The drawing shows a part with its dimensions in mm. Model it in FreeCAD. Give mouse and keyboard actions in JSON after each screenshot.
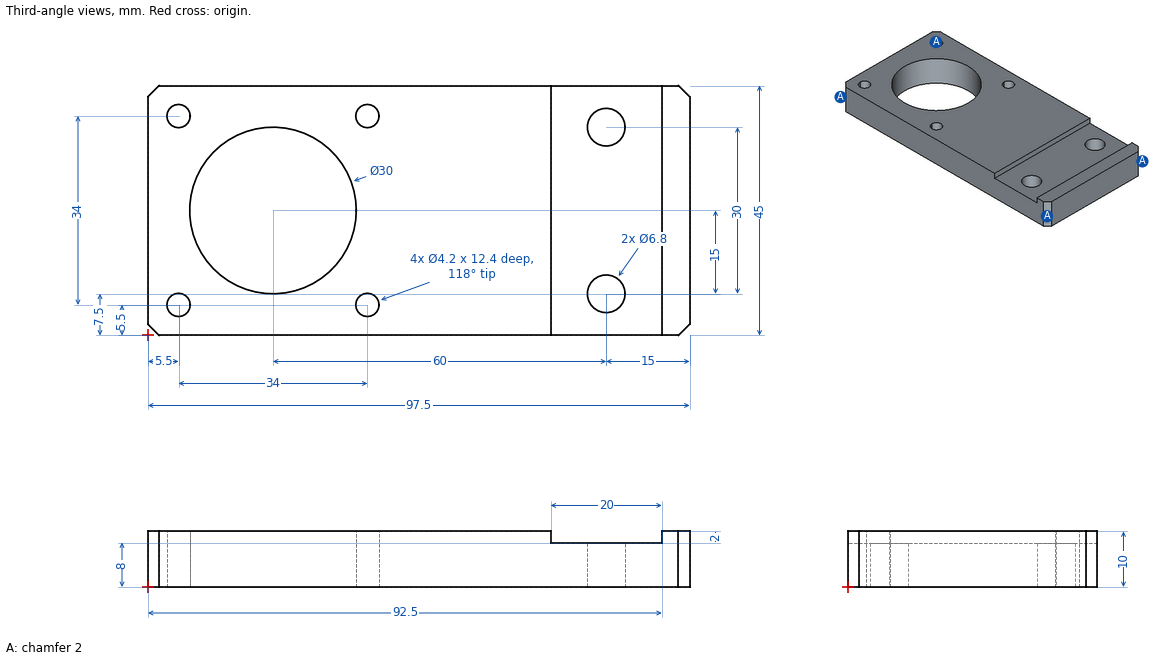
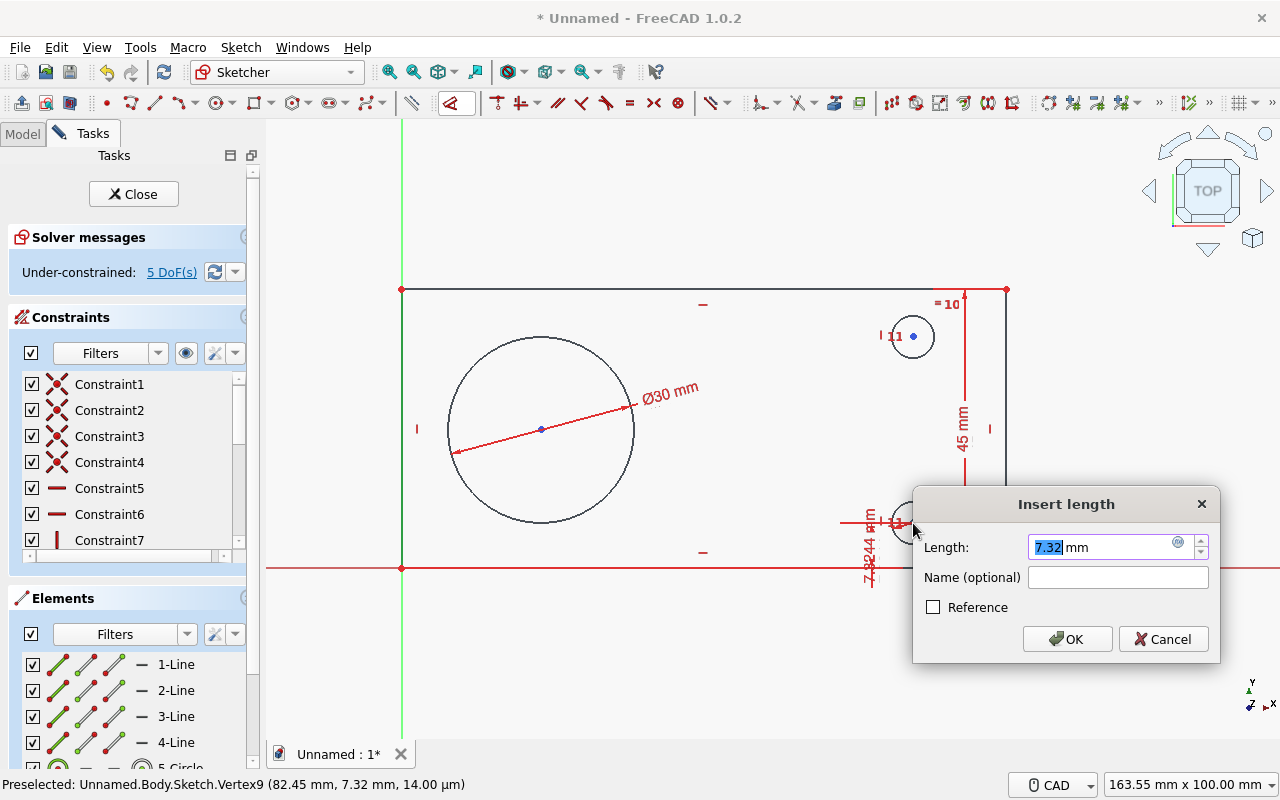
{"action": "type", "text": "7.5"}
{"action": "key", "text": "Return"}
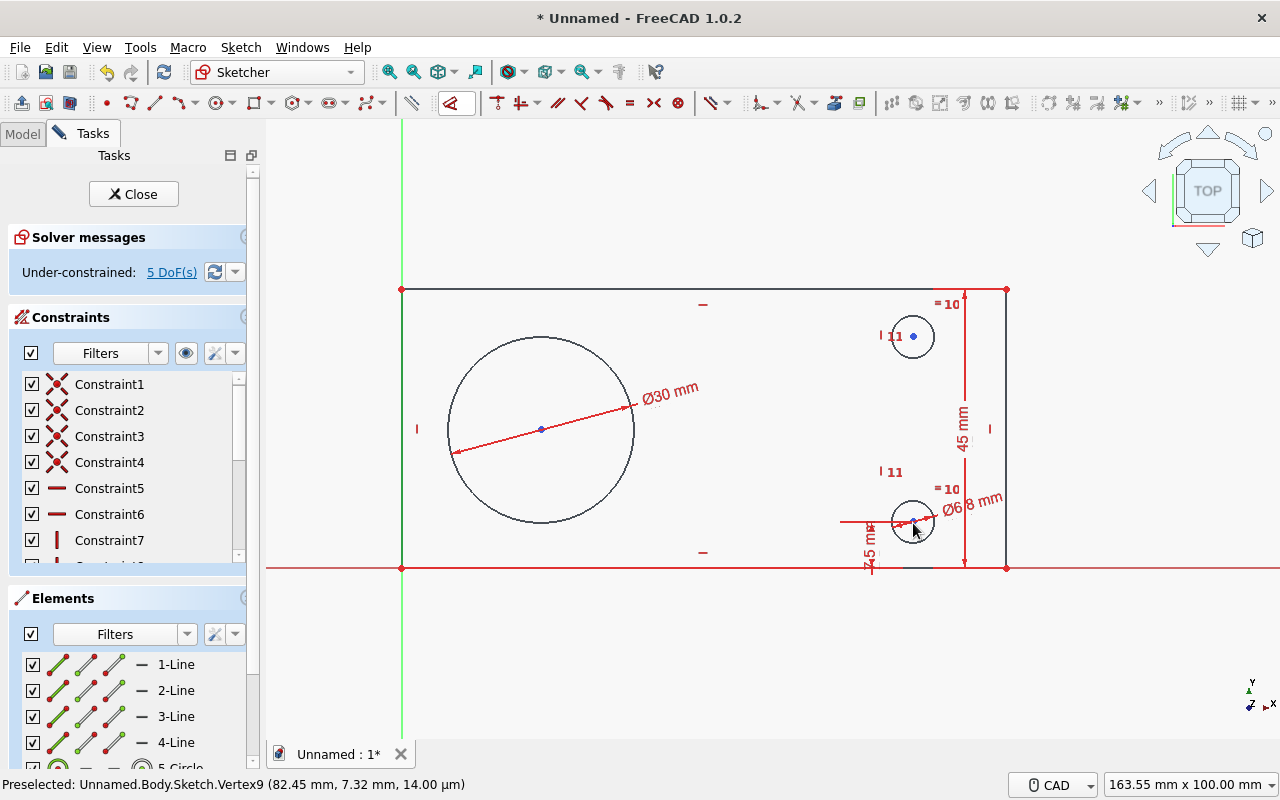
{"action": "left_click", "coordinate": [1006, 568]}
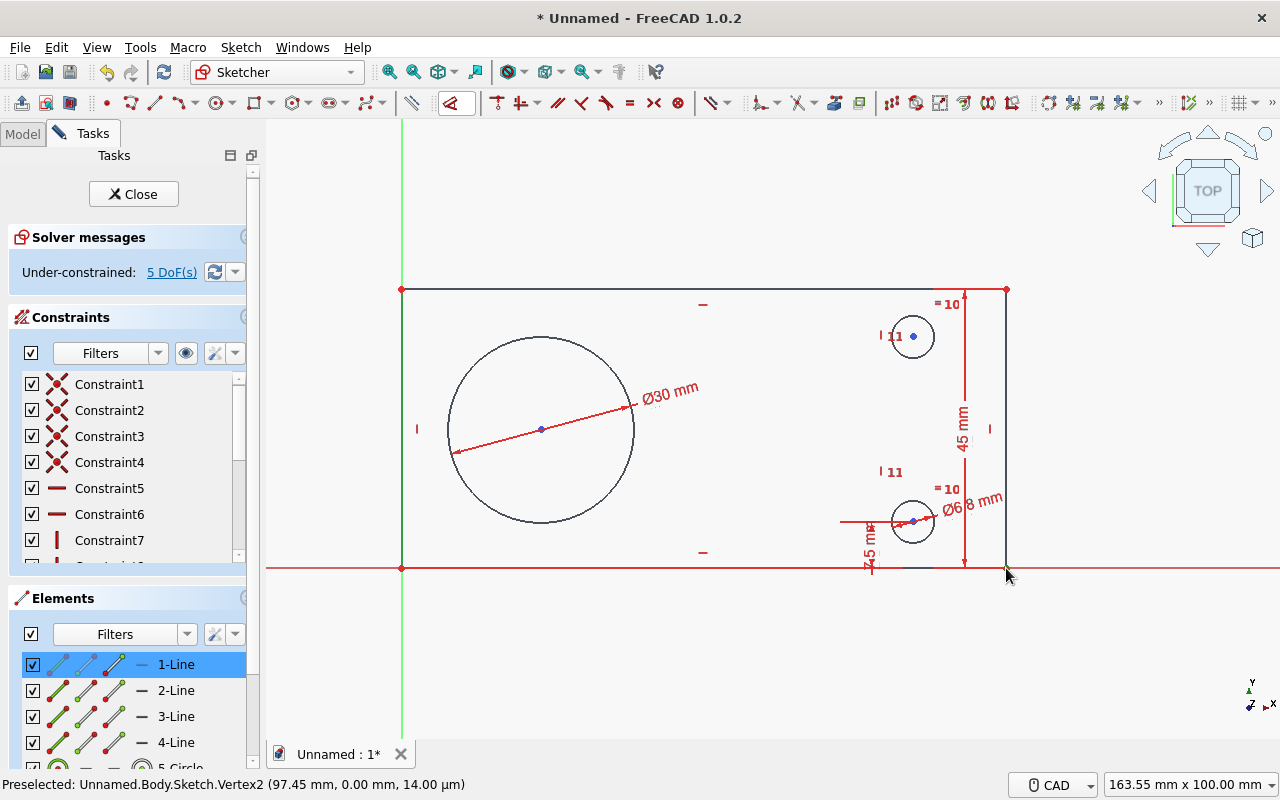
{"action": "left_click", "coordinate": [913, 522]}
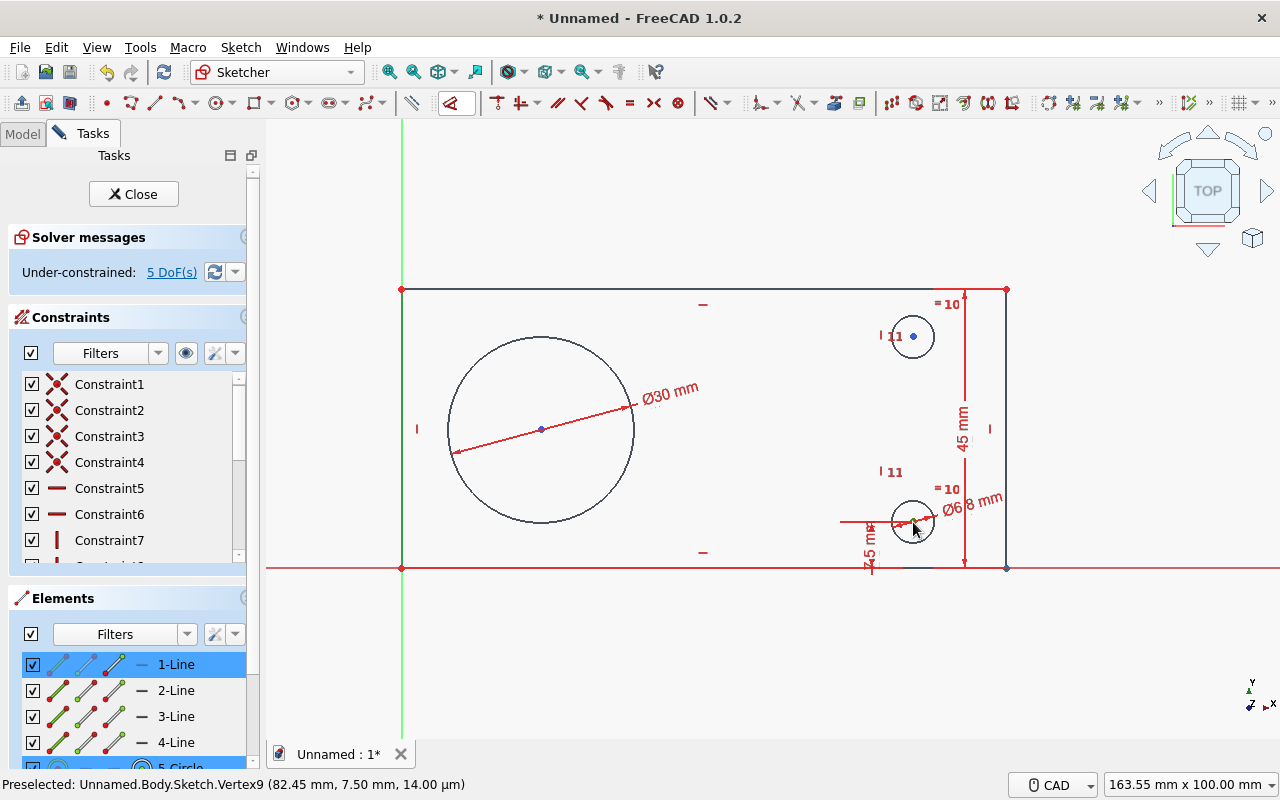
{"action": "key", "text": "l"}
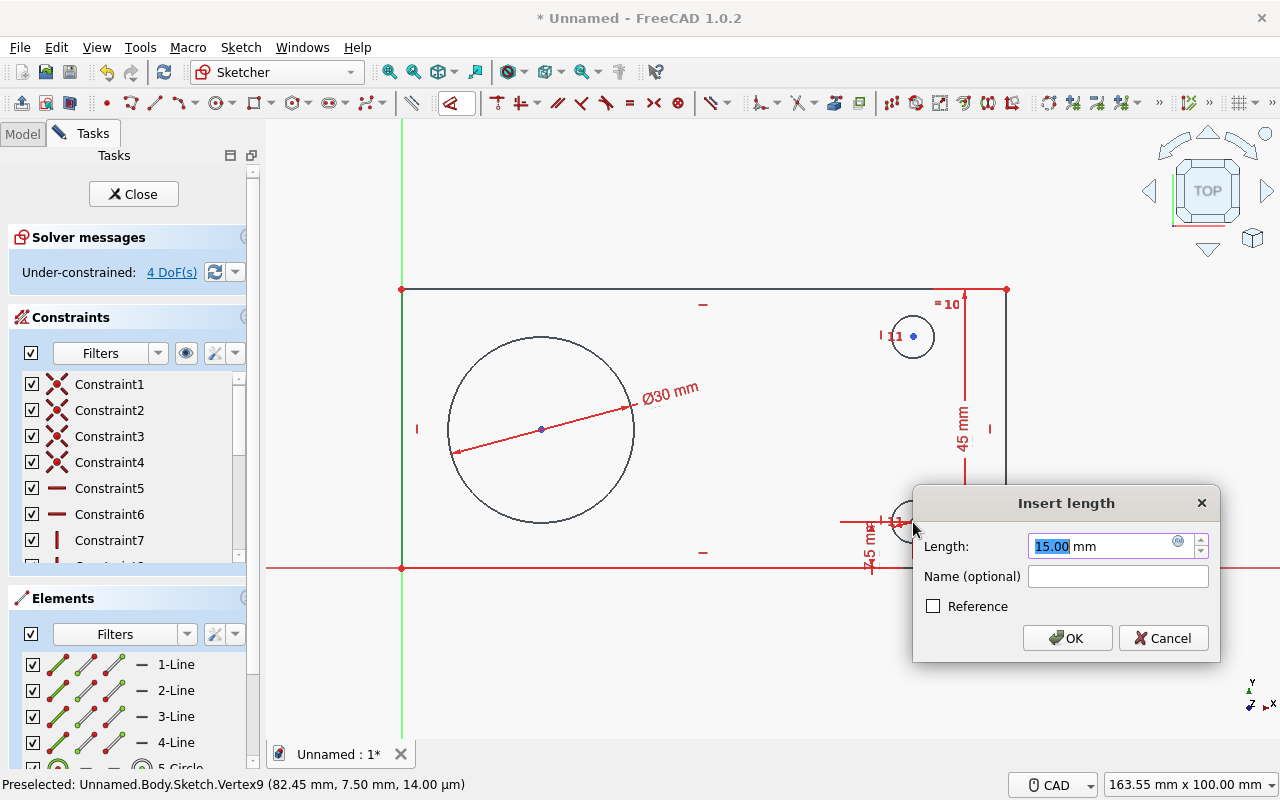
{"action": "type", "text": "15"}
{"action": "key", "text": "Return"}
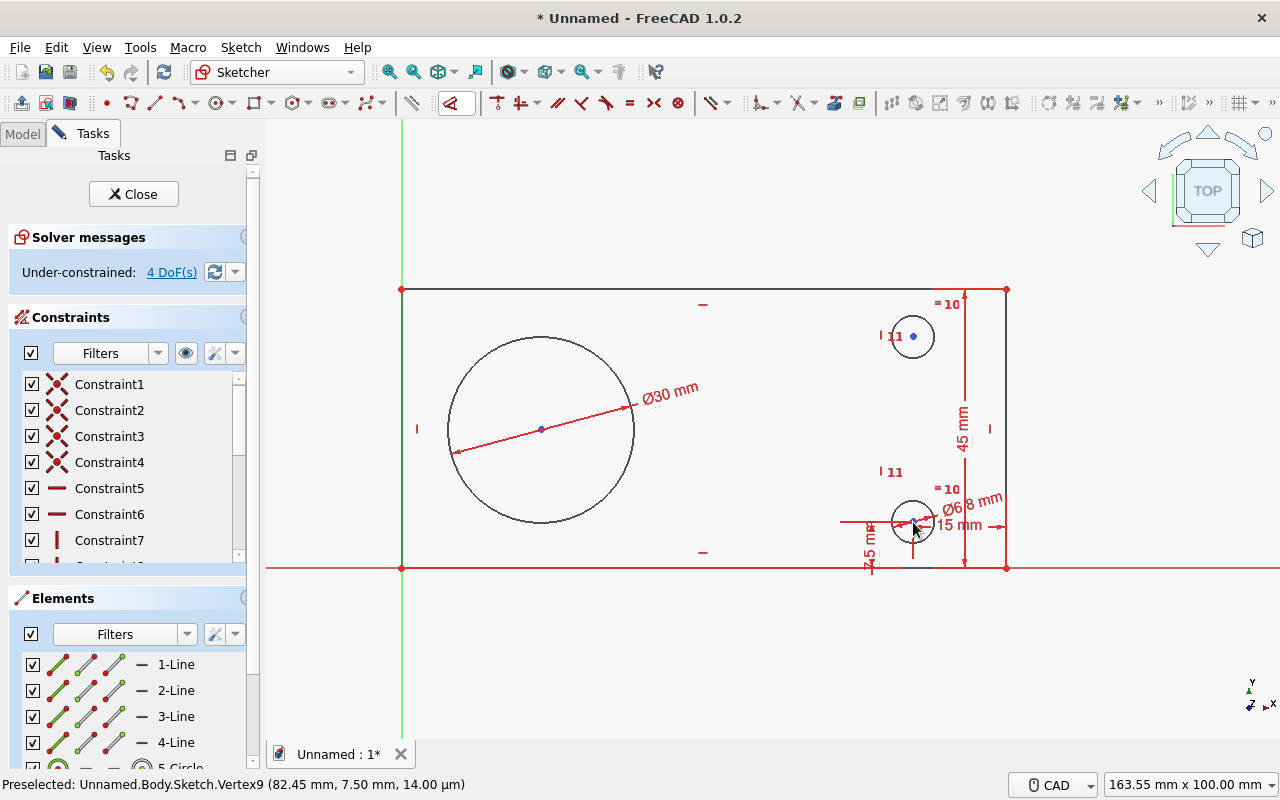
{"action": "left_click", "coordinate": [913, 522]}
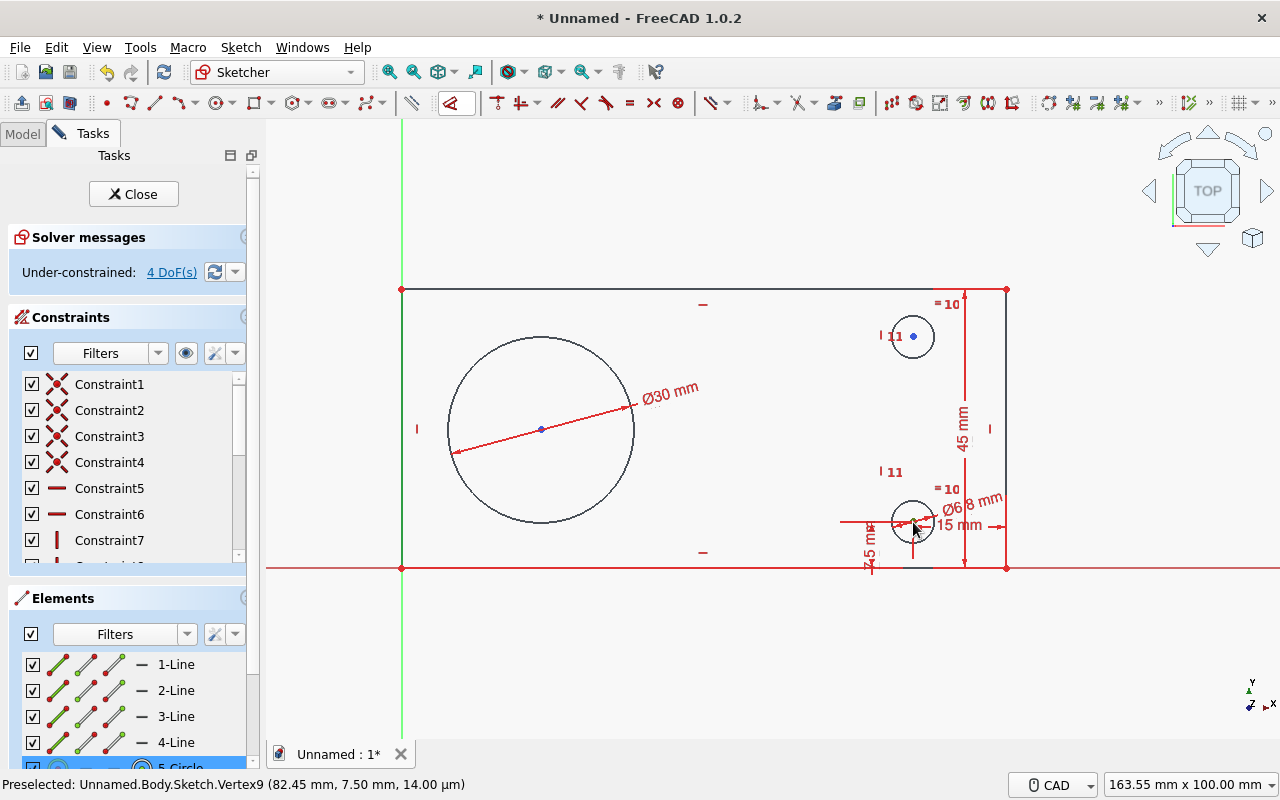
{"action": "left_click", "coordinate": [541, 430]}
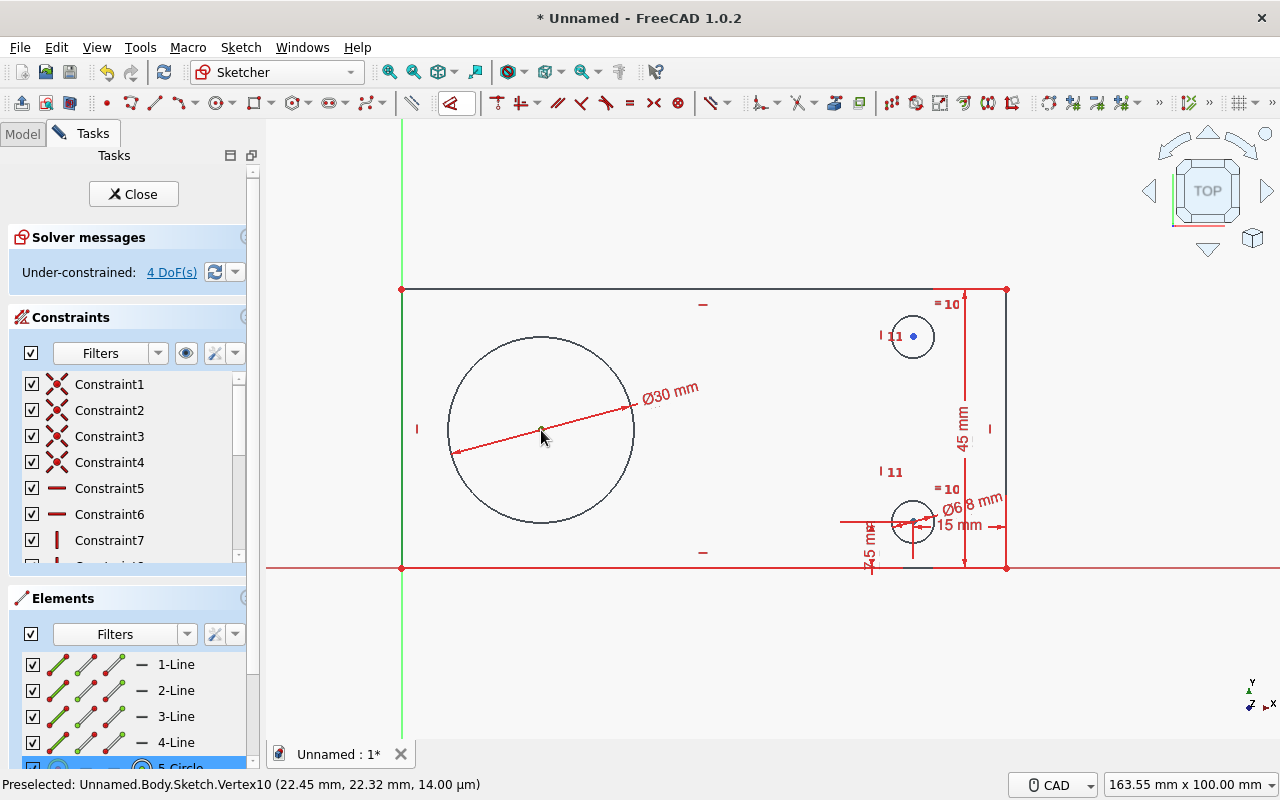
{"action": "left_click", "coordinate": [470, 104]}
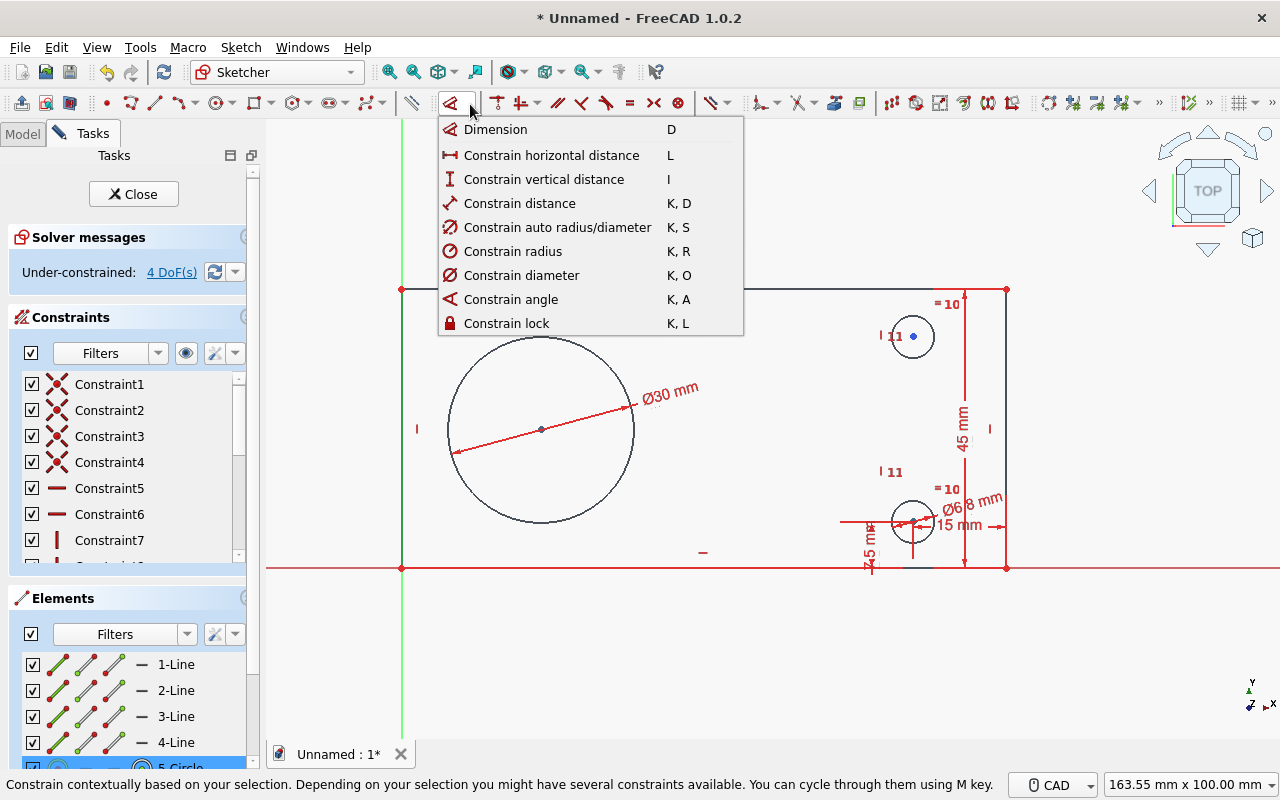
{"action": "left_click", "coordinate": [591, 155]}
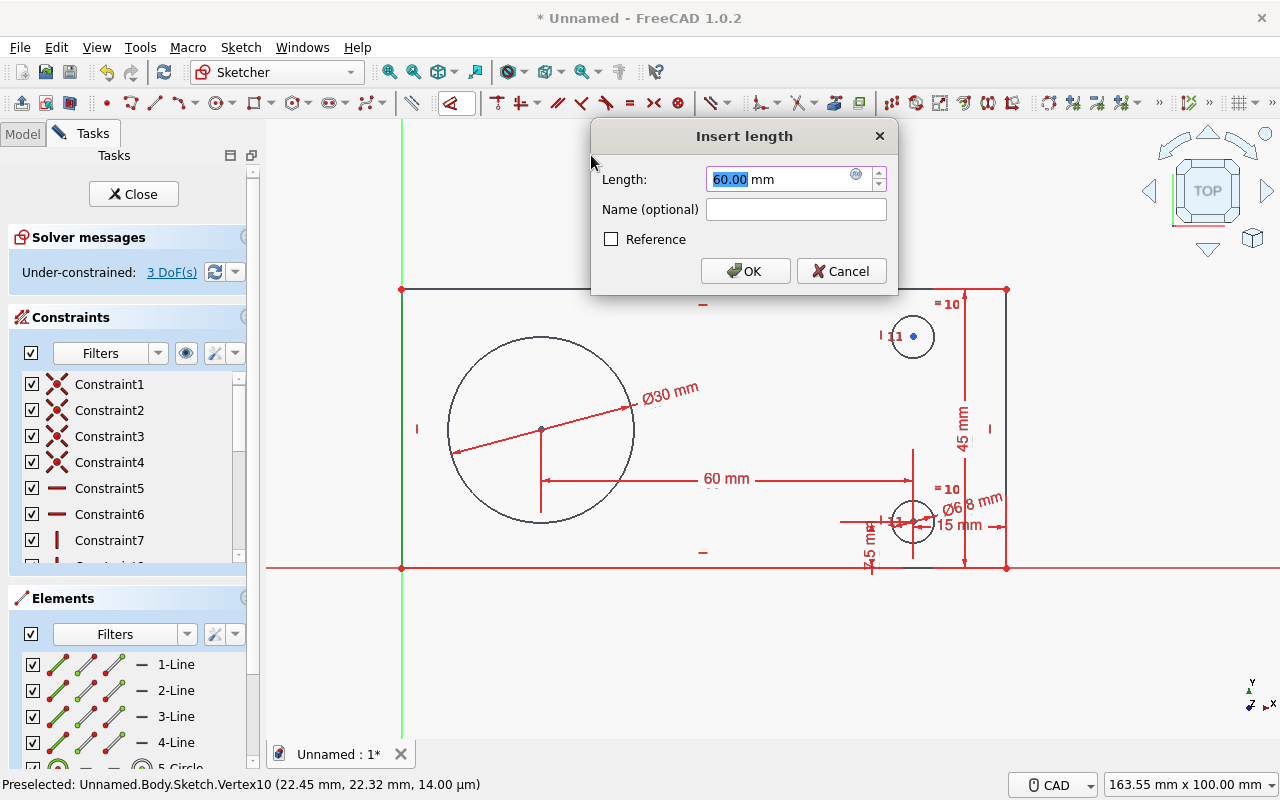
{"action": "type", "text": "60"}
{"action": "key", "text": "Return"}